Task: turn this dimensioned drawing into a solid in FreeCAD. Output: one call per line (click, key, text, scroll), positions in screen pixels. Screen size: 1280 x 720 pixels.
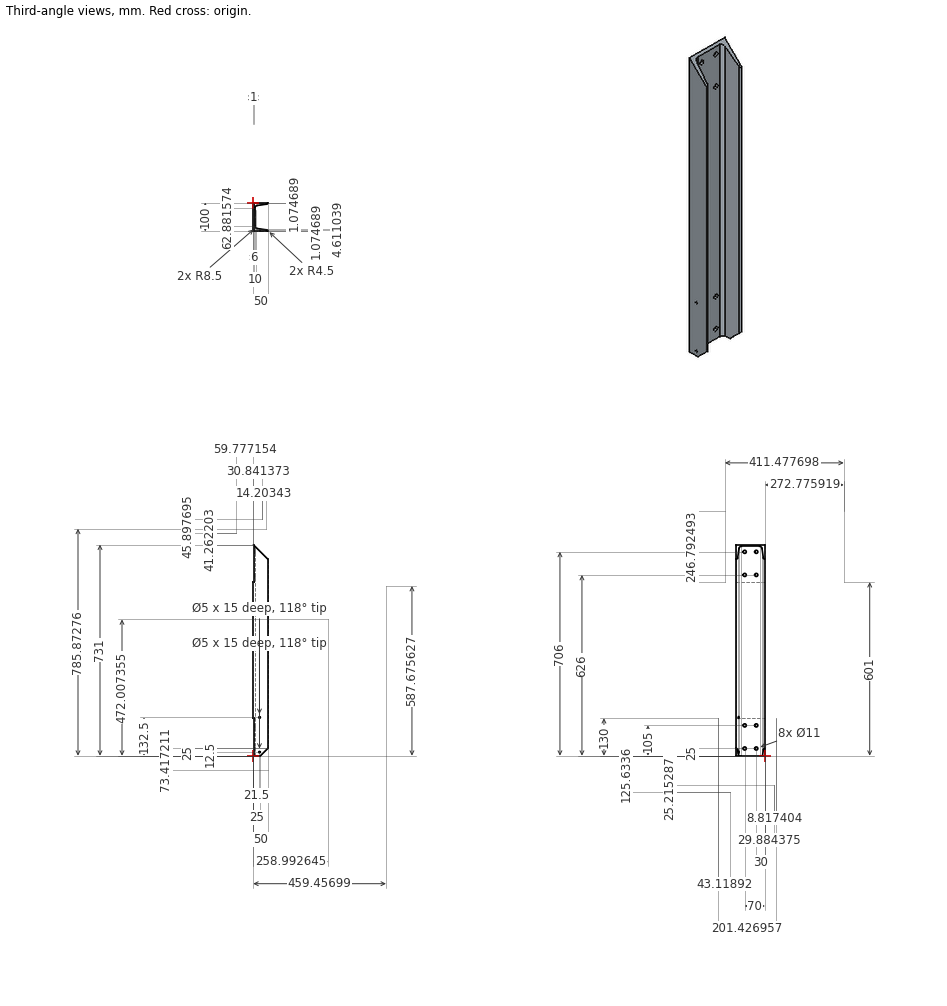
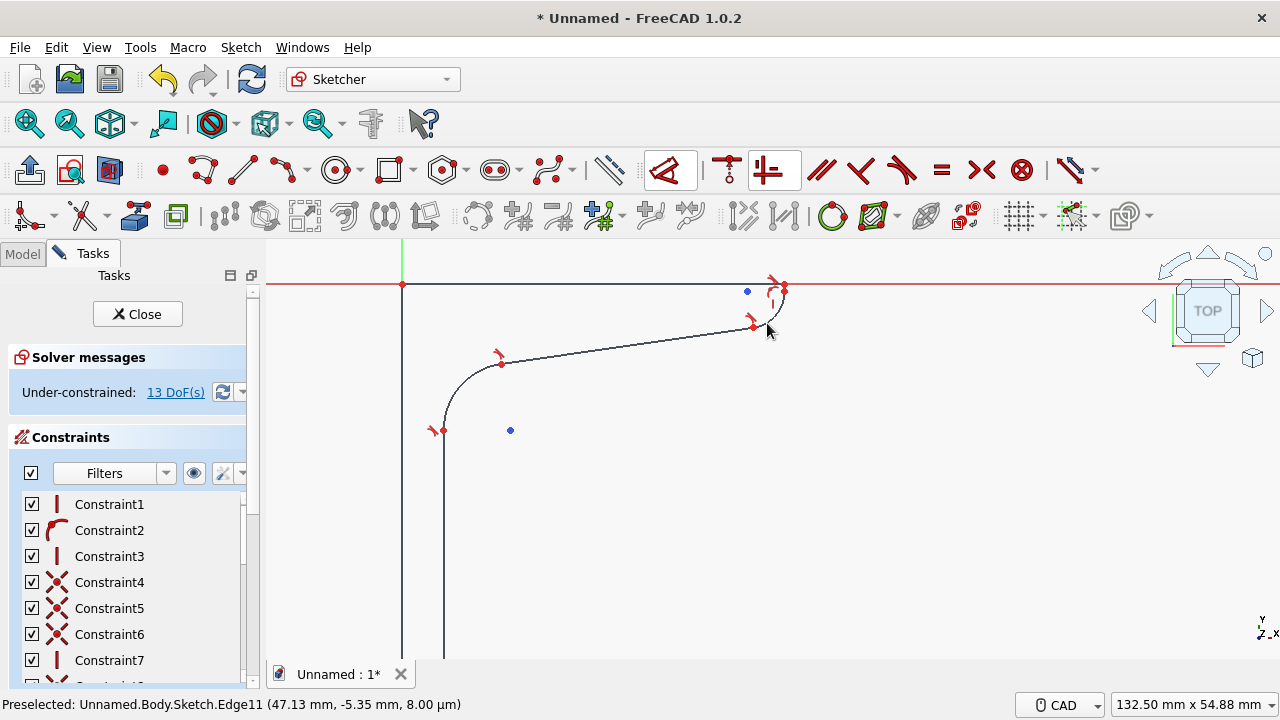
scroll(769, 322, down, 5)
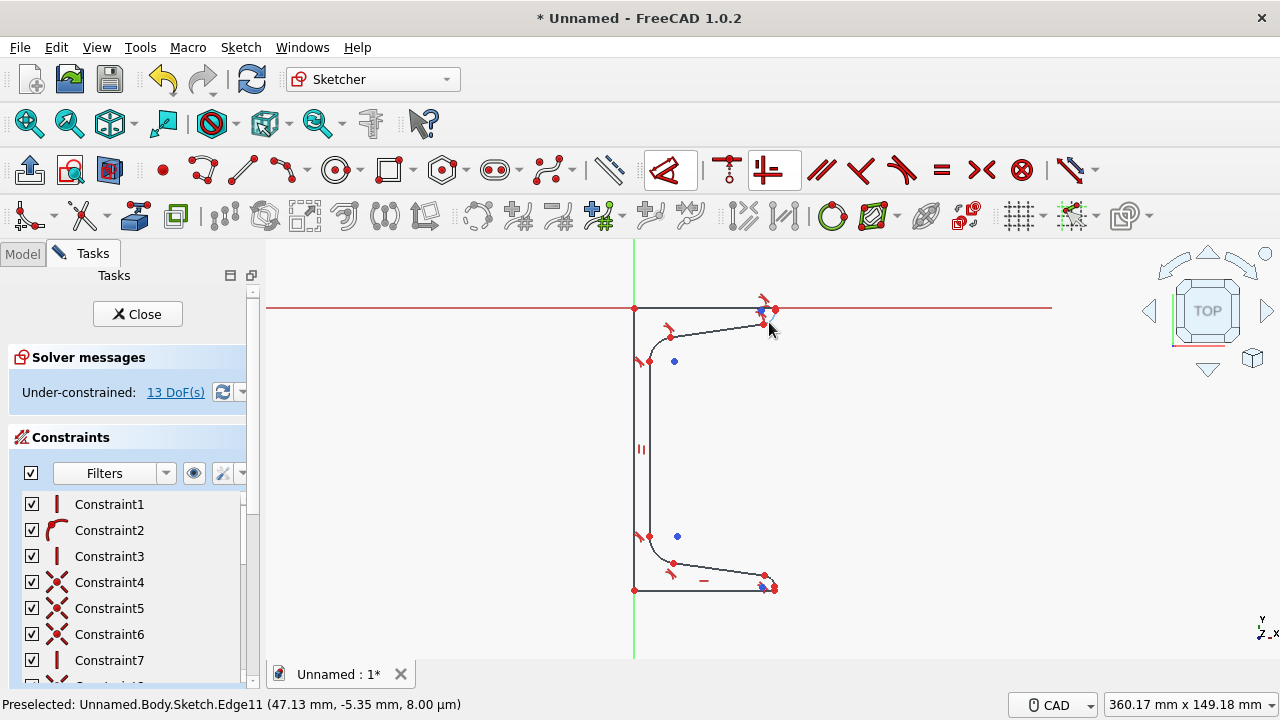
scroll(775, 589, up, 10)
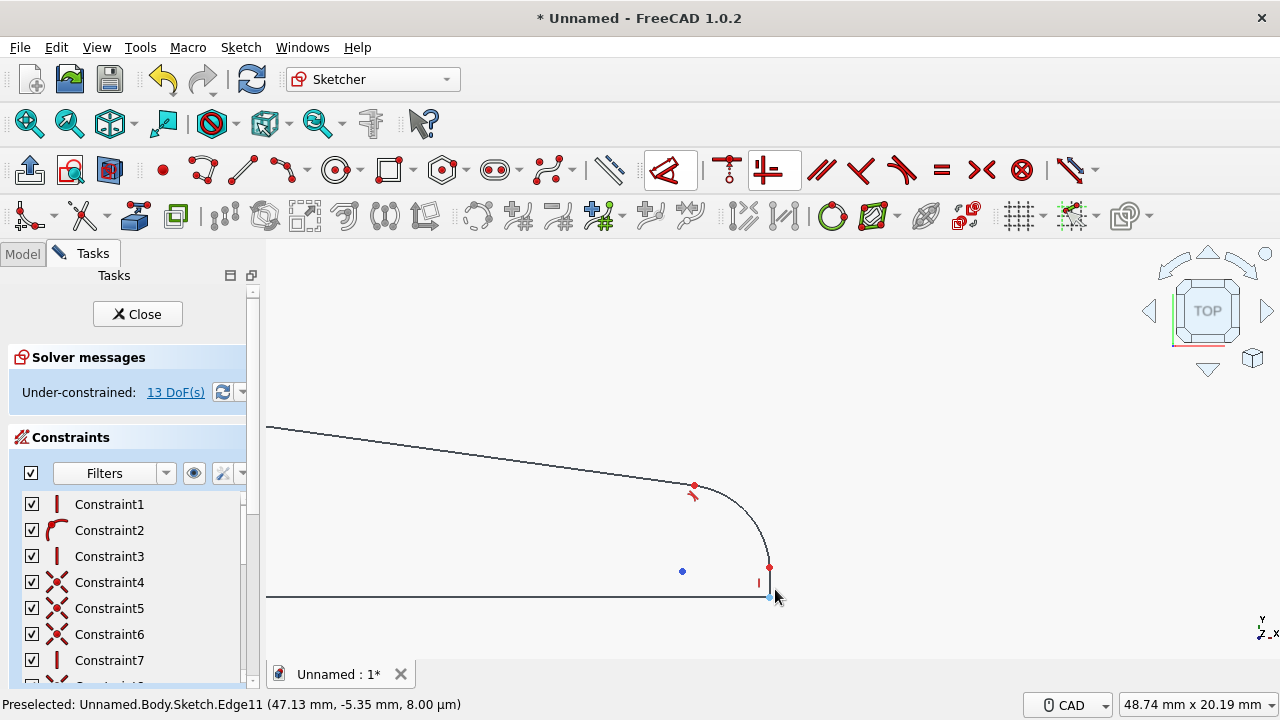
click(770, 582)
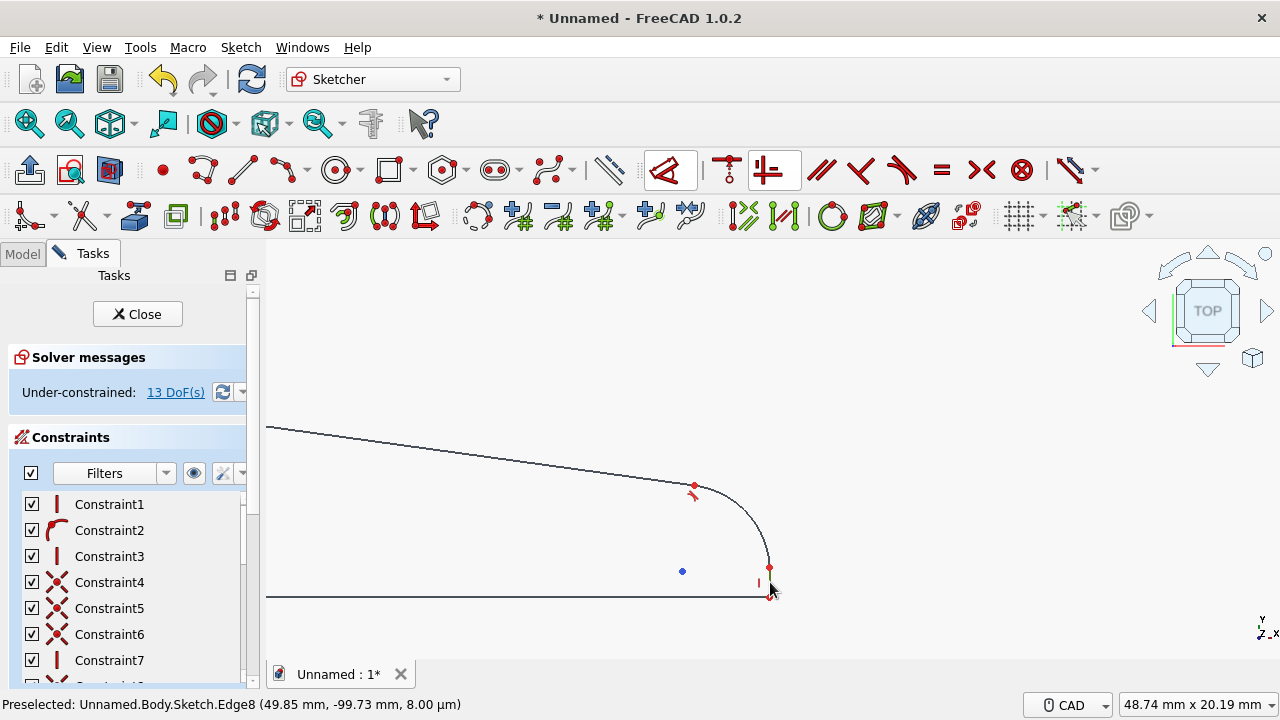
click(761, 533)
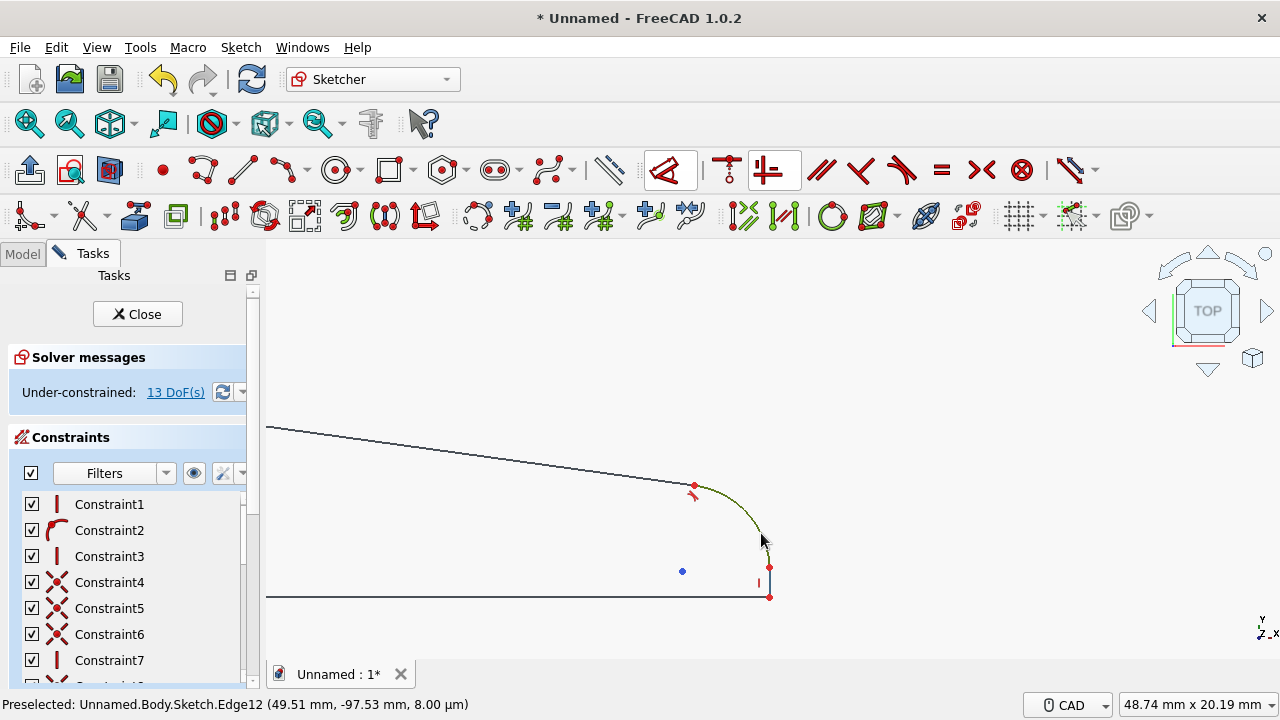
key(t)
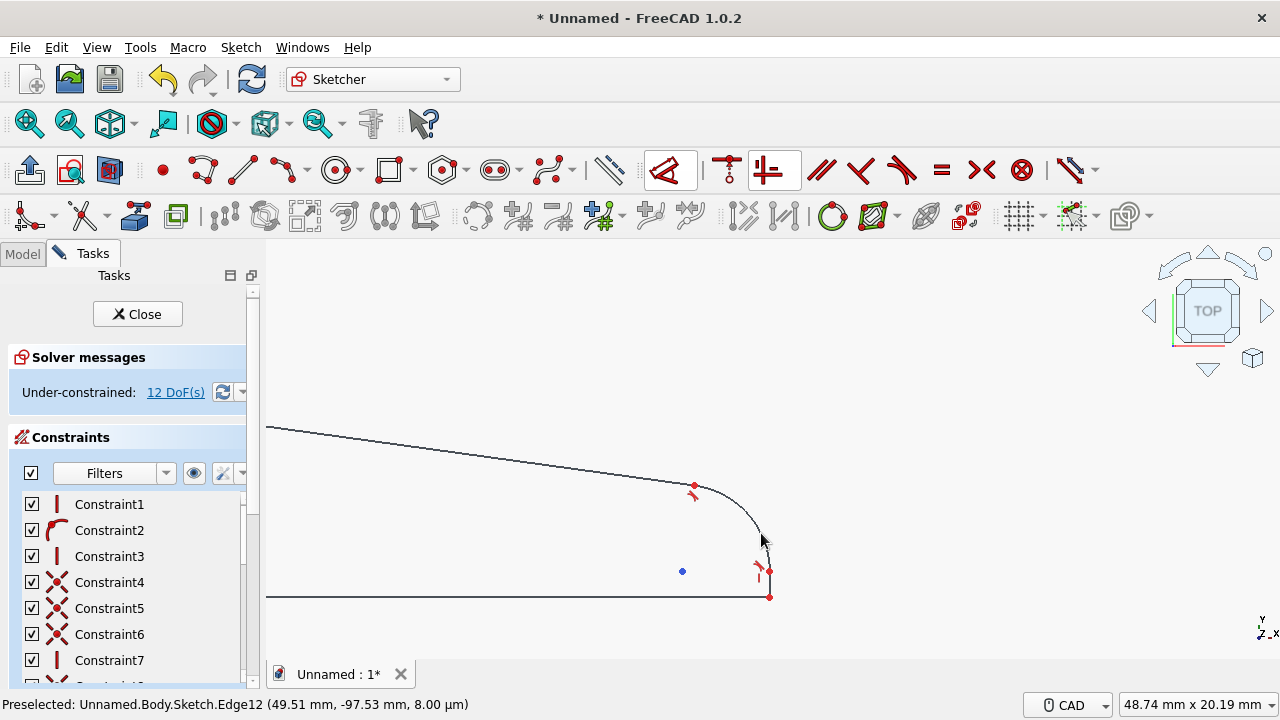
scroll(775, 590, down, 10)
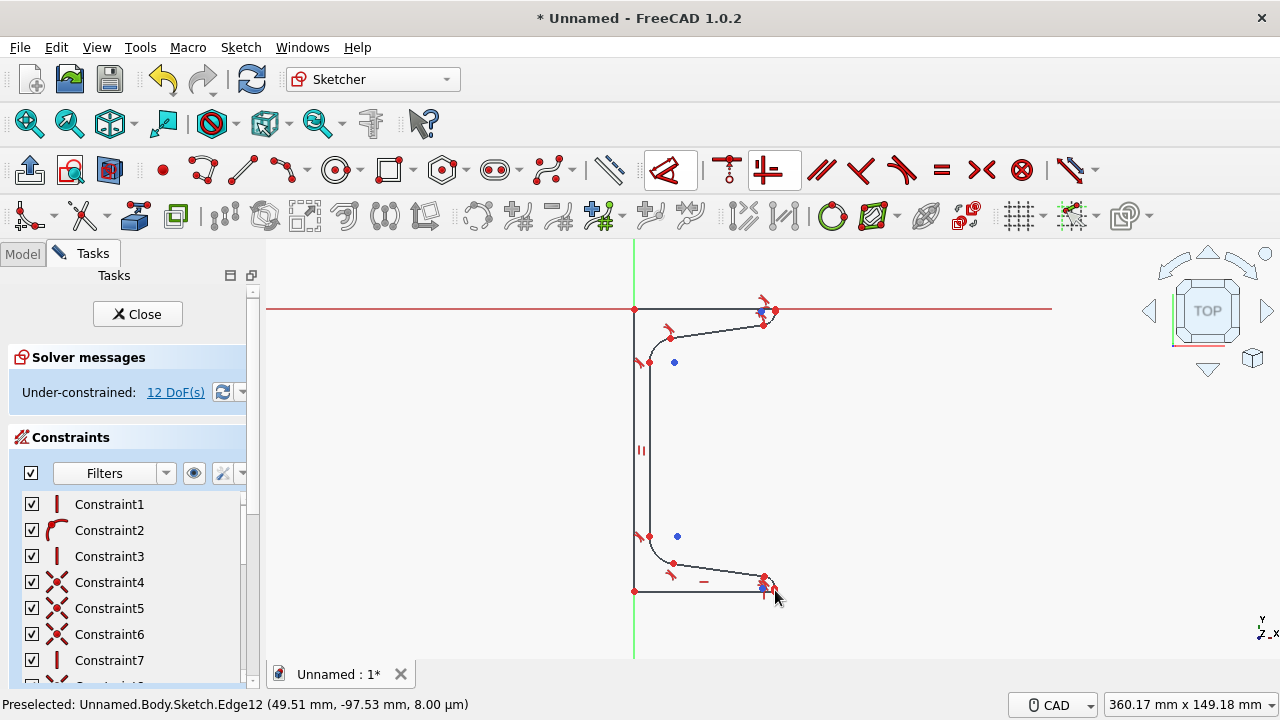
click(652, 548)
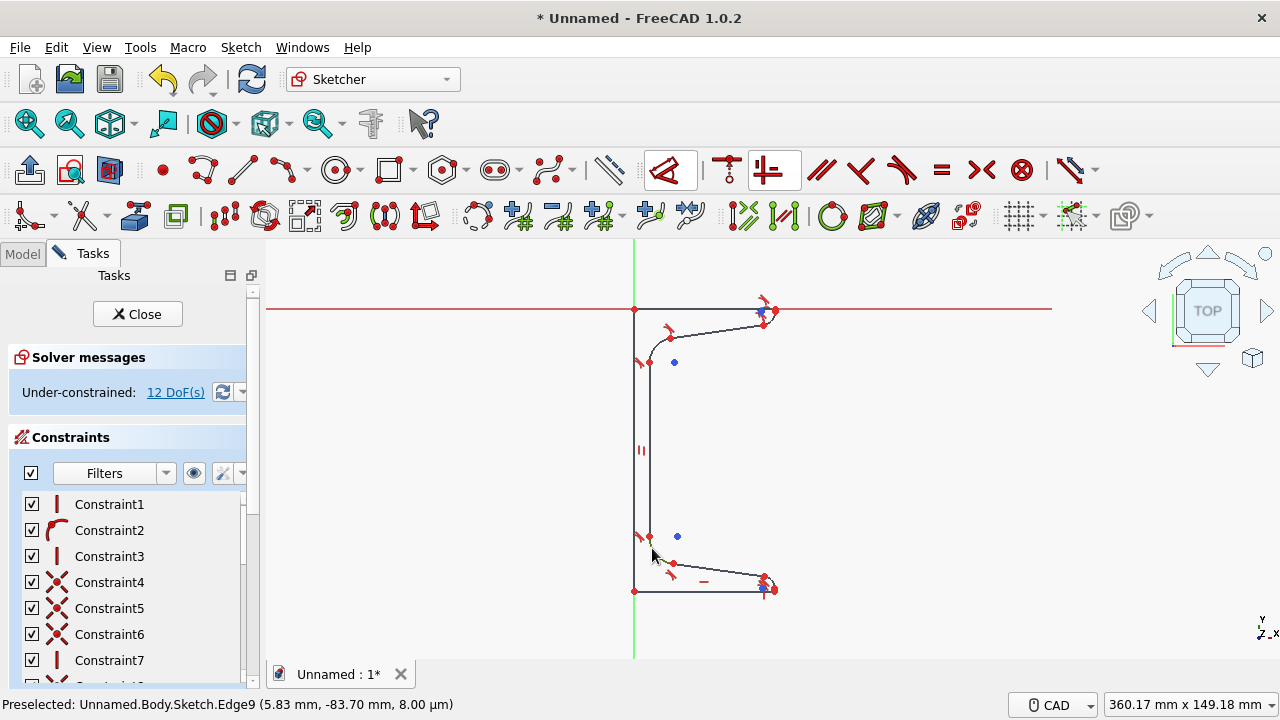
scroll(661, 342, up, 2)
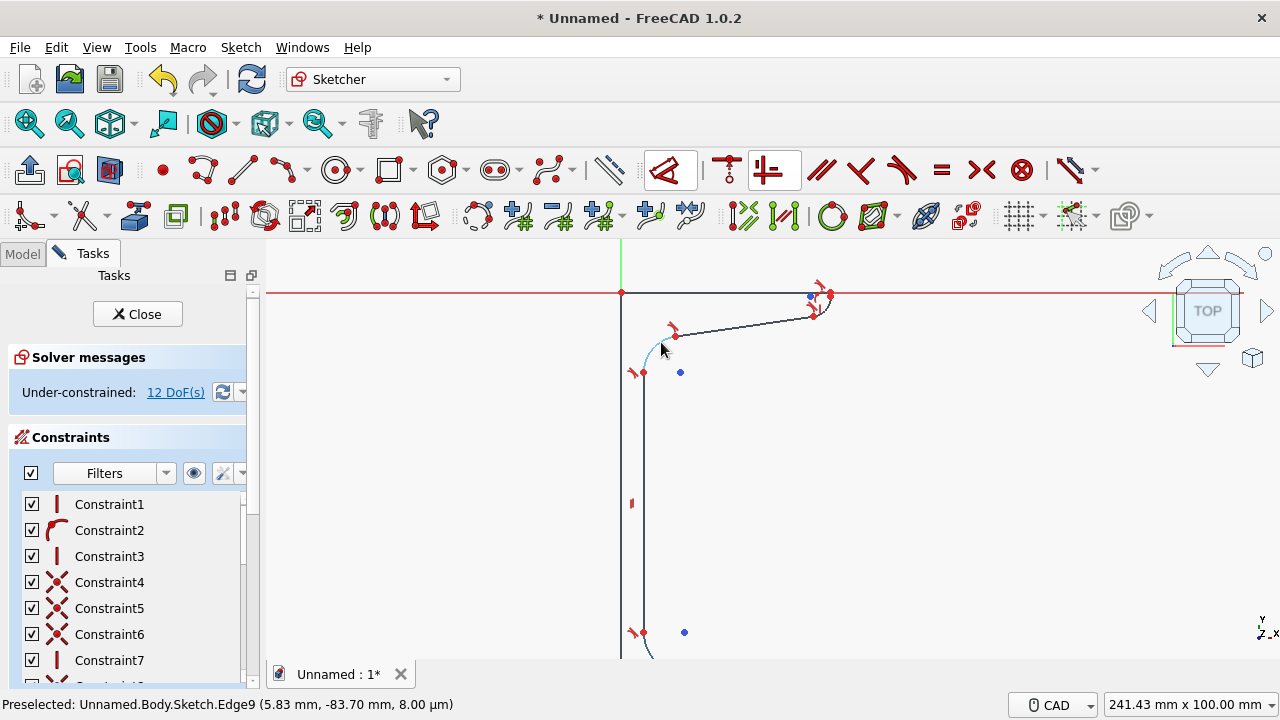
click(661, 342)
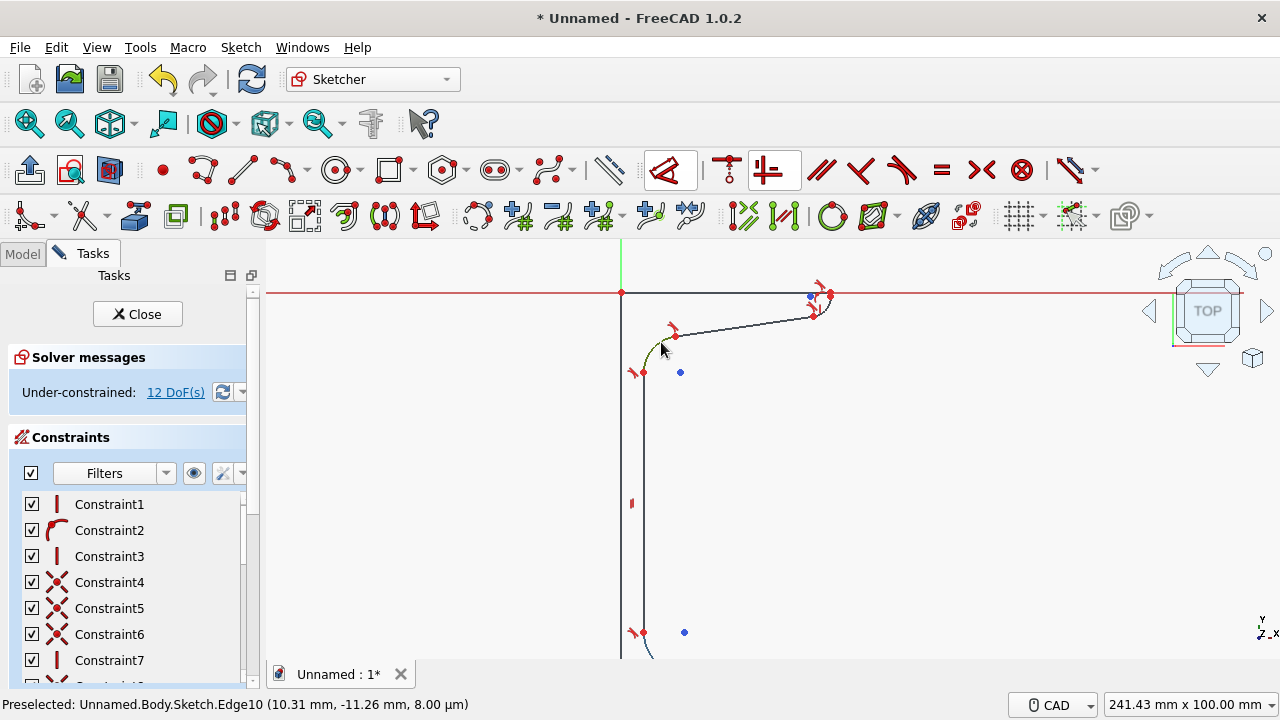
click(942, 170)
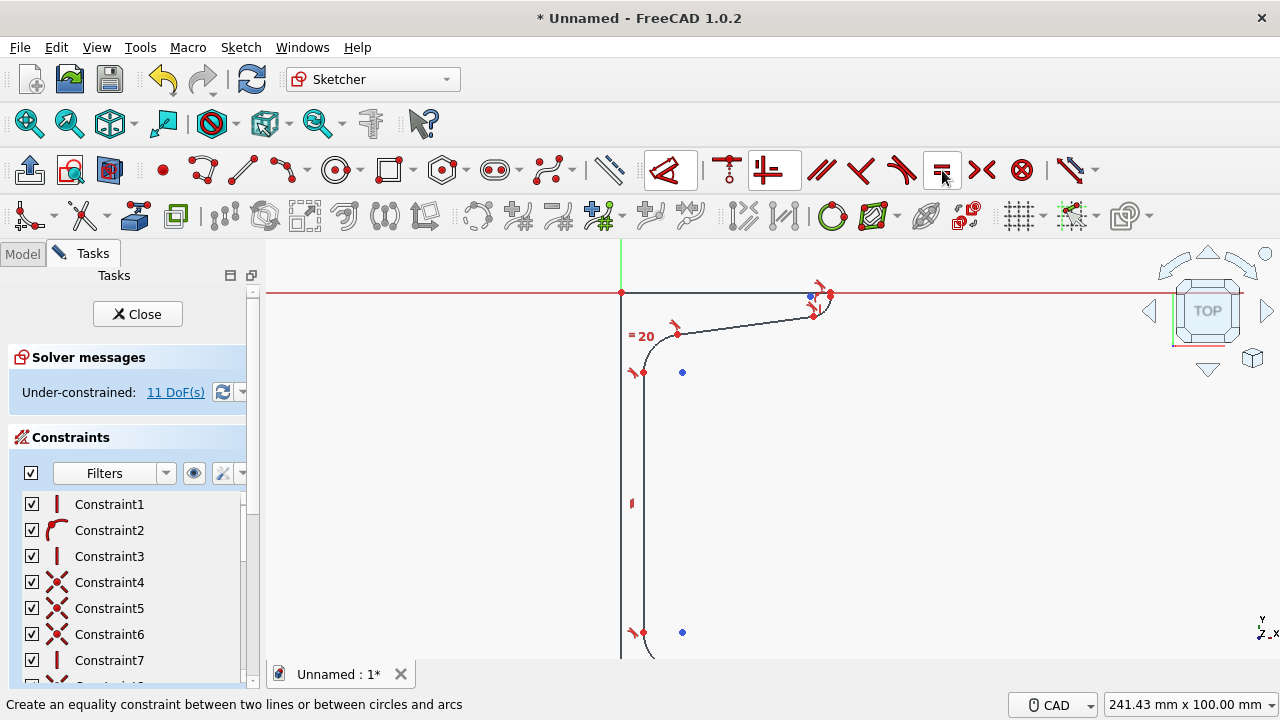
click(822, 314)